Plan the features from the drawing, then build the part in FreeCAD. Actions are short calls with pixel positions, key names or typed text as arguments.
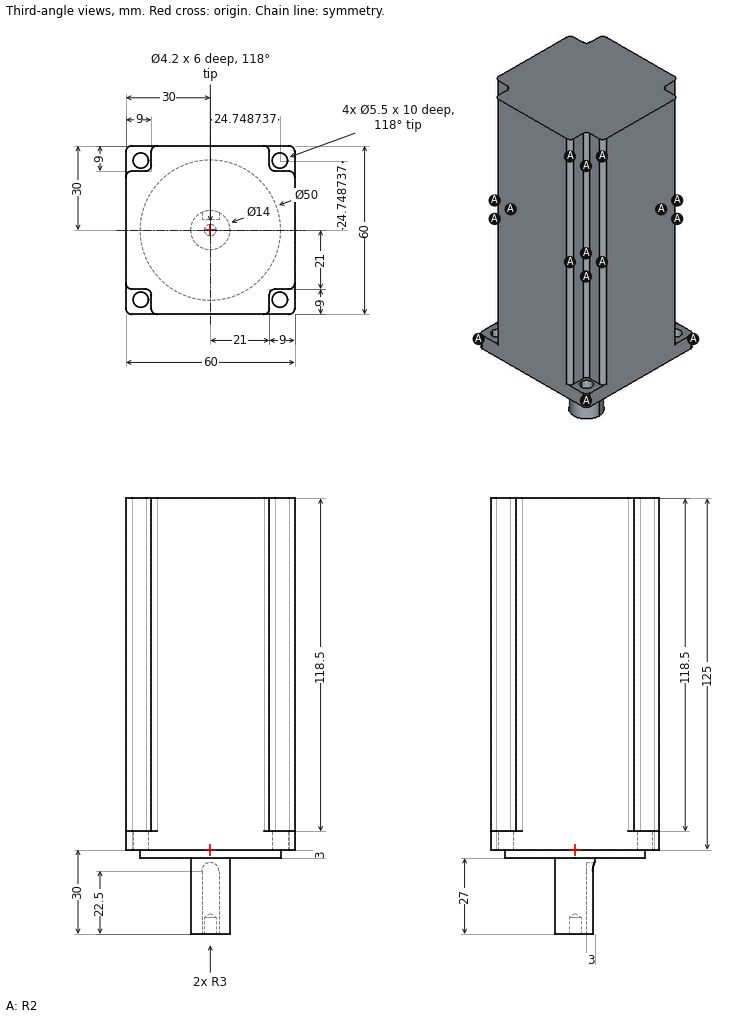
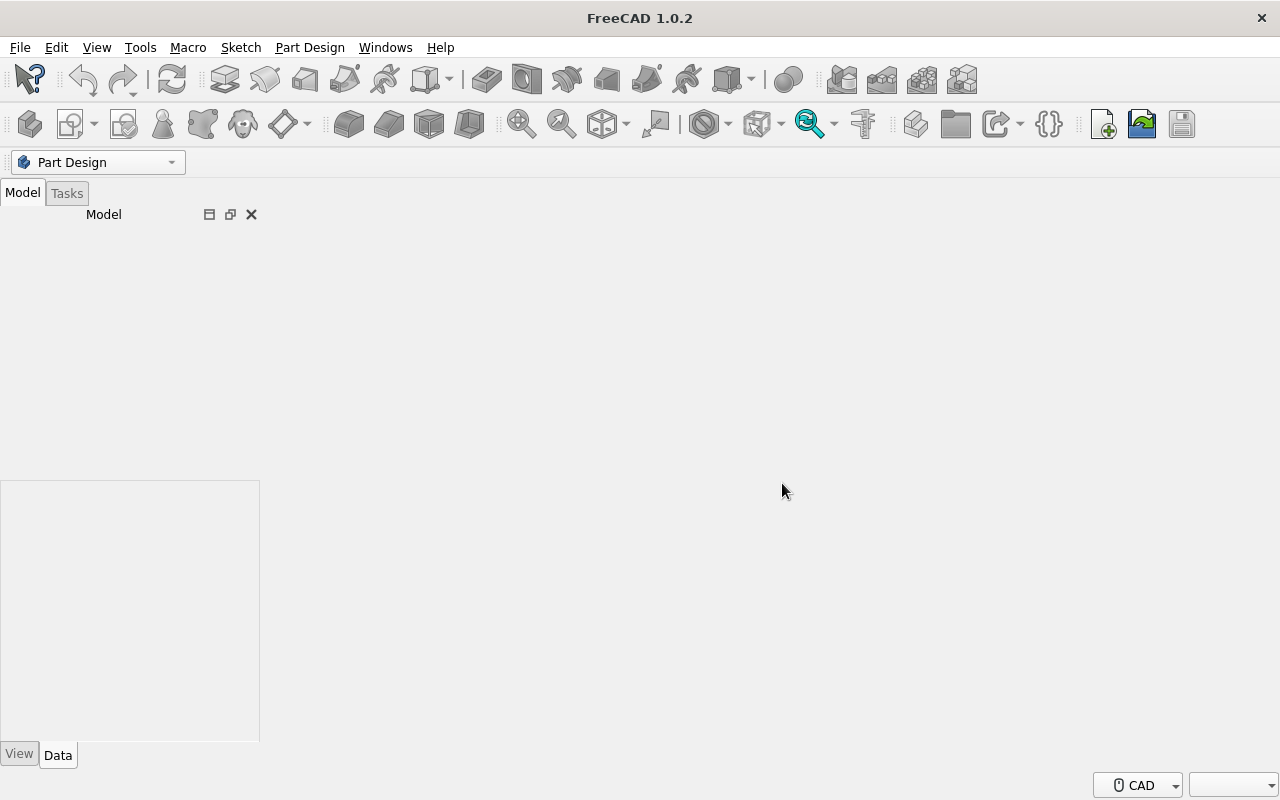
click(1102, 124)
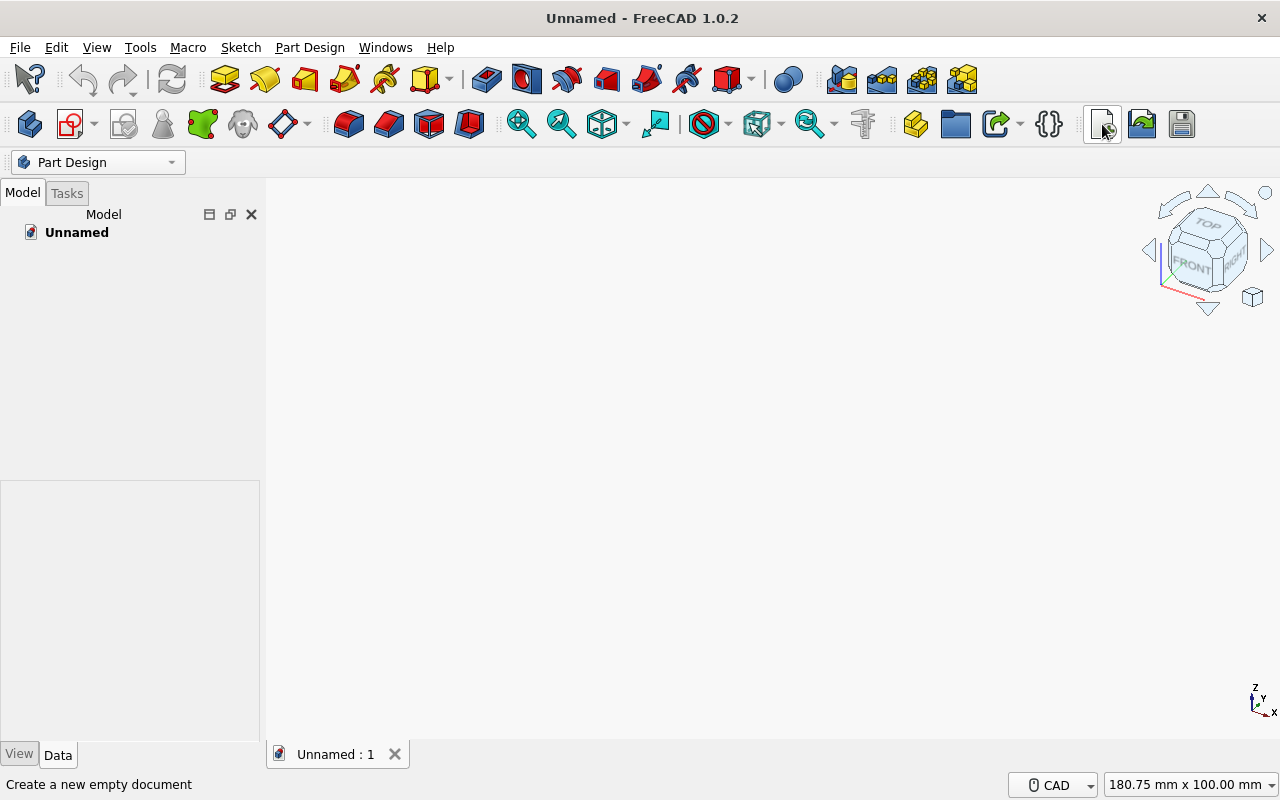
click(70, 124)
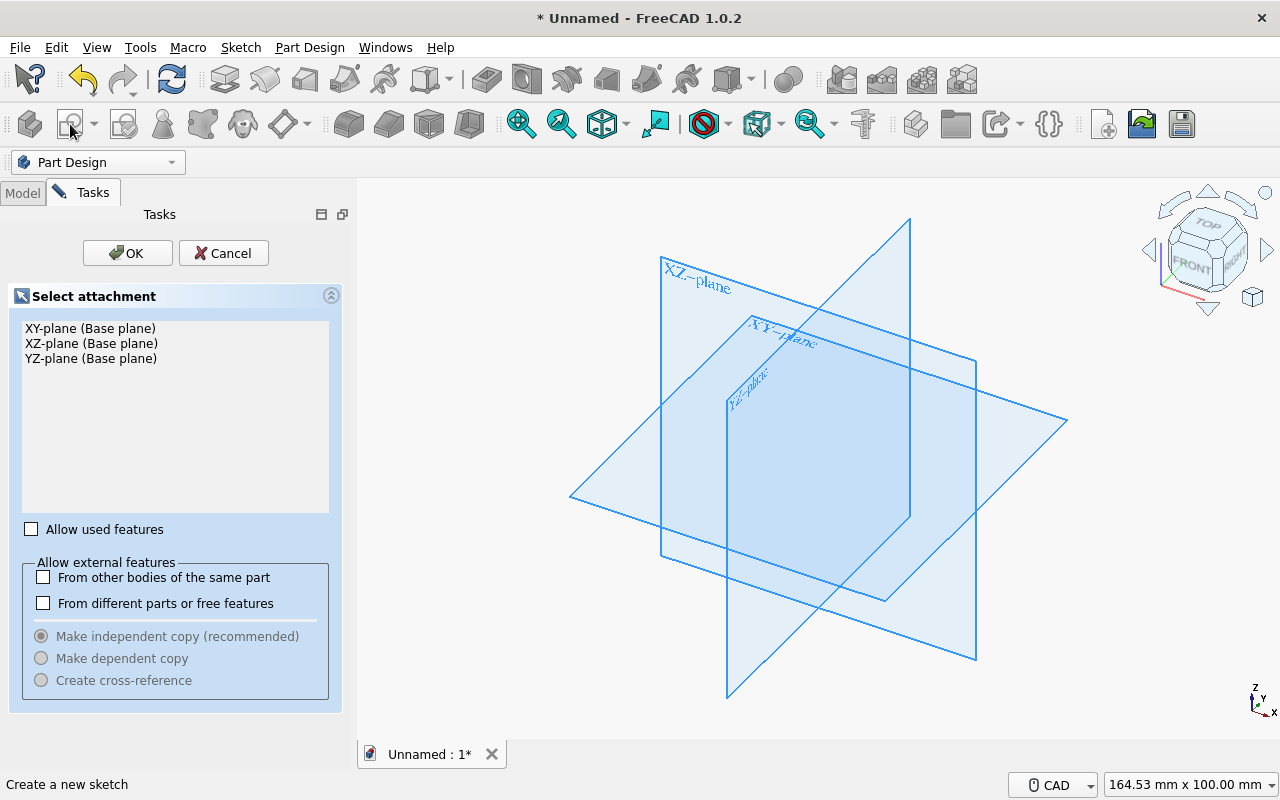
click(82, 328)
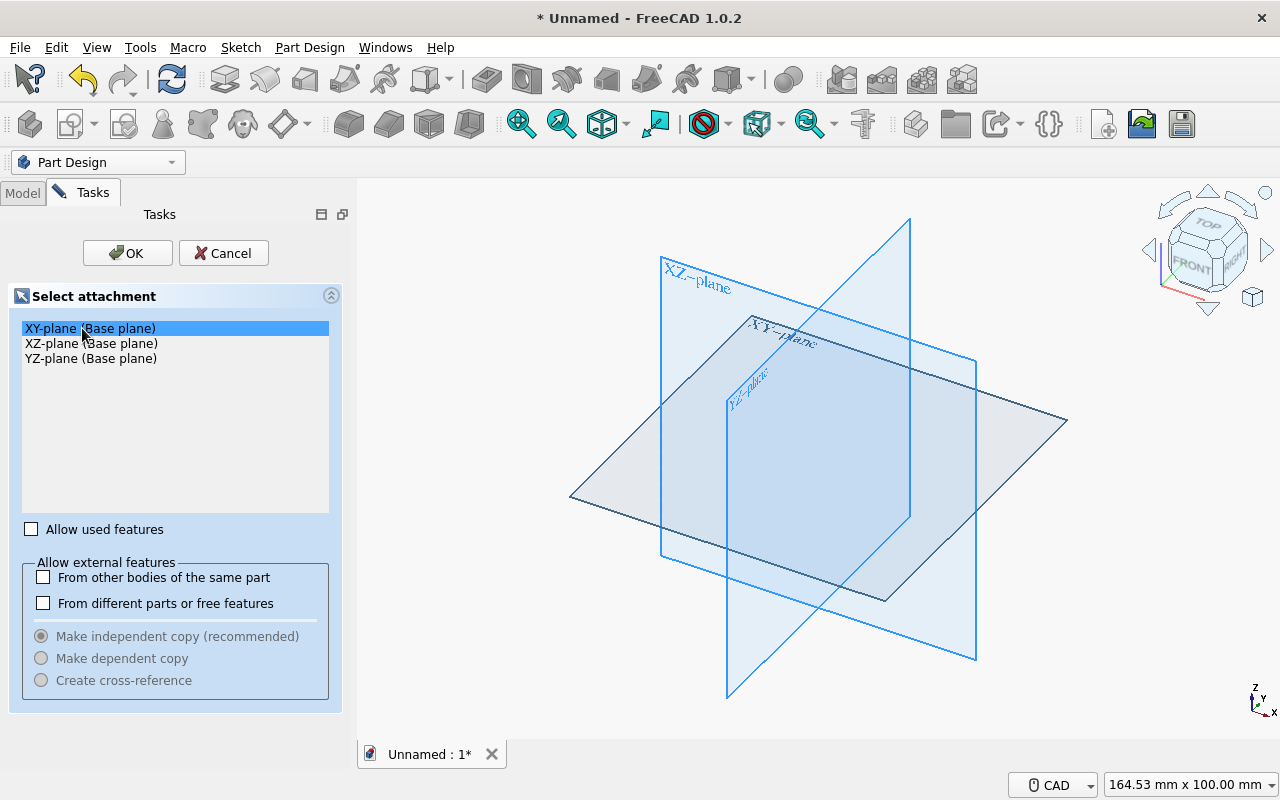
click(128, 253)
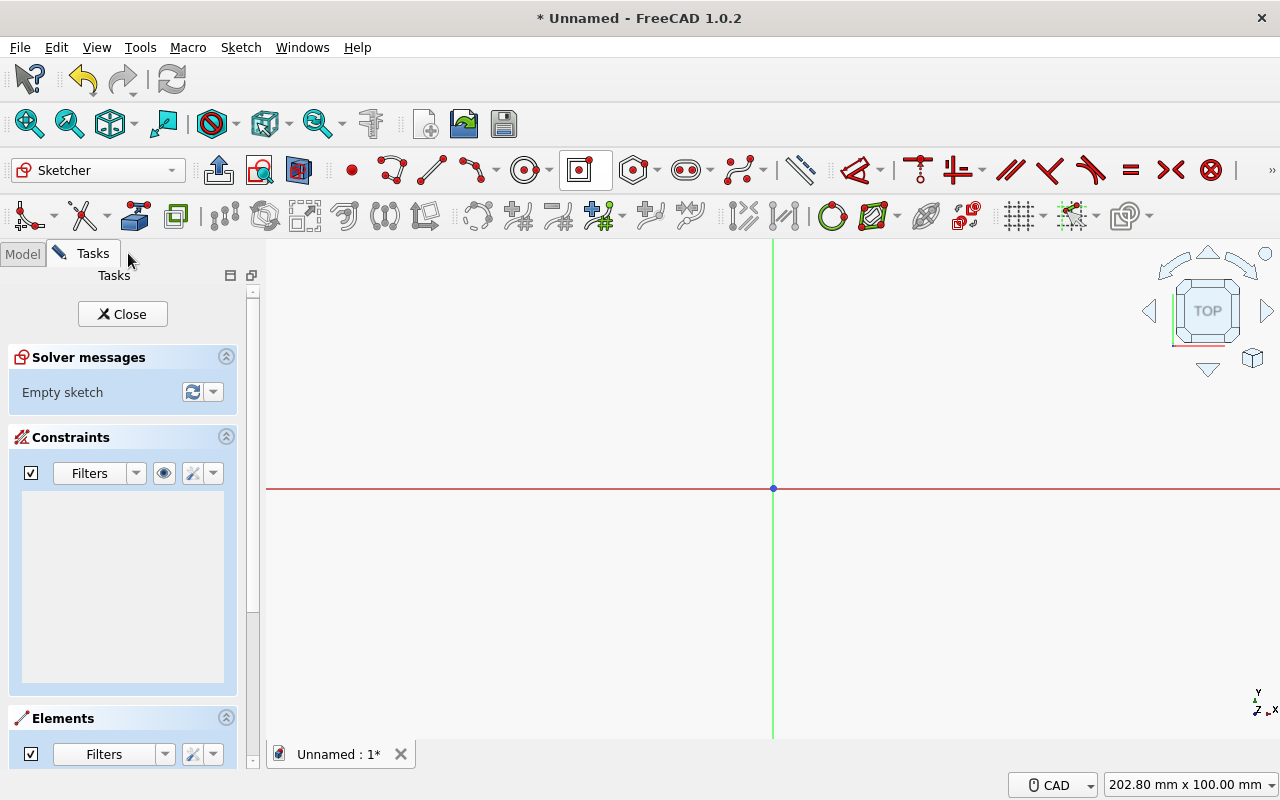
key(g)
key(v)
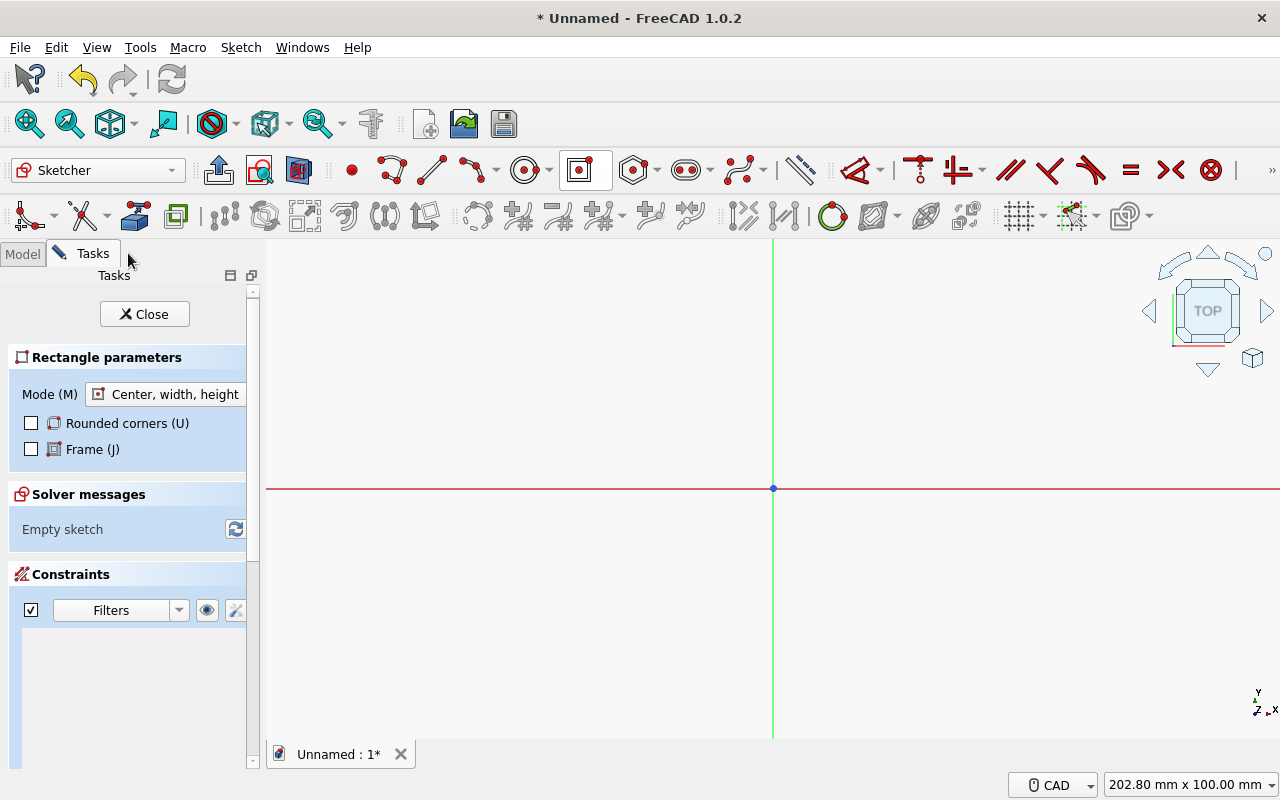
click(773, 489)
move(923, 339)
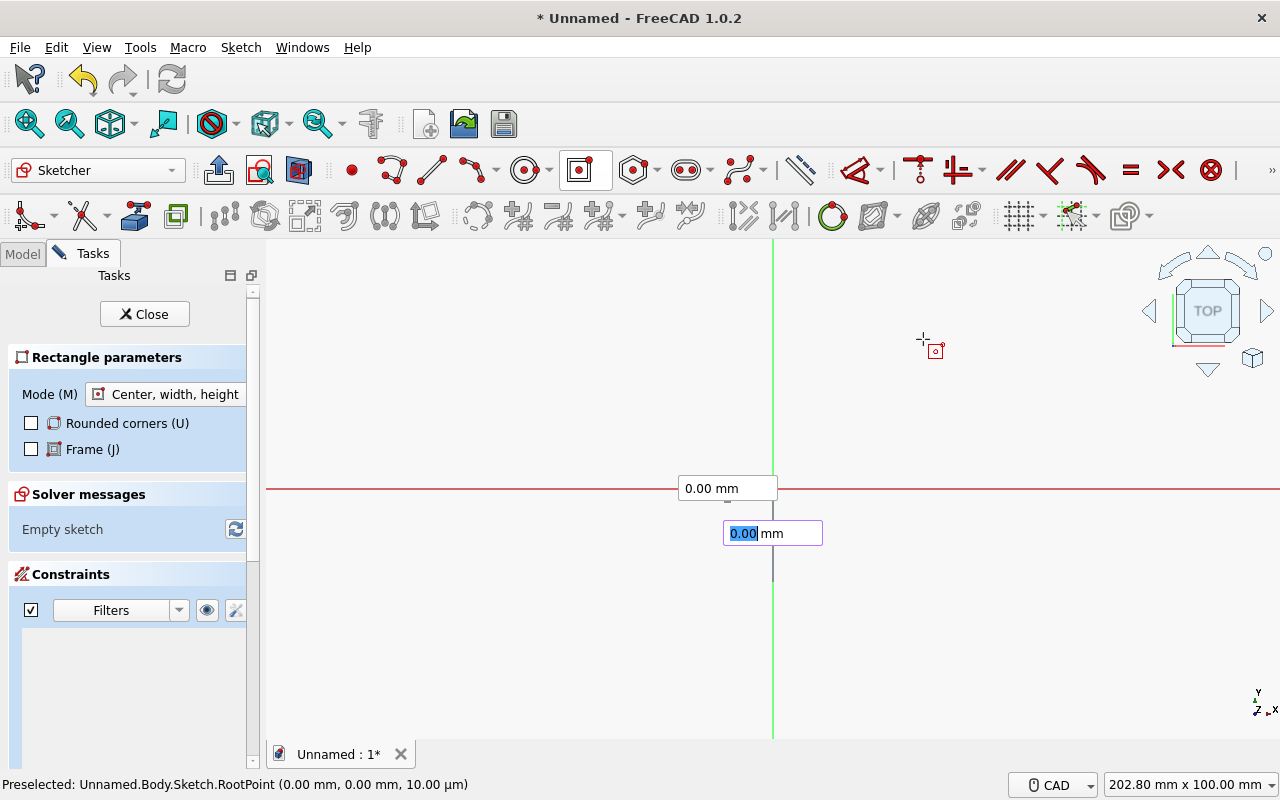
text(60)
key(Tab)
text(60)
key(Return)
key(Escape)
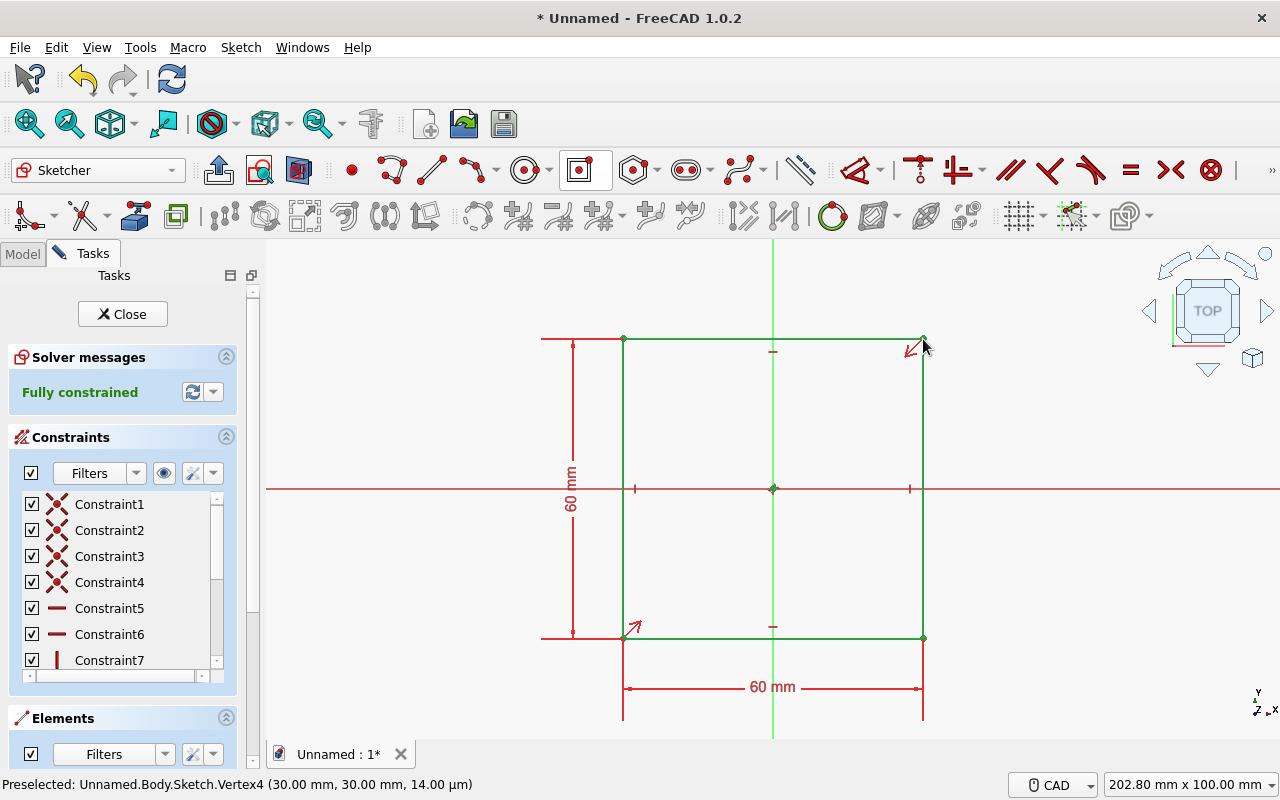
click(123, 314)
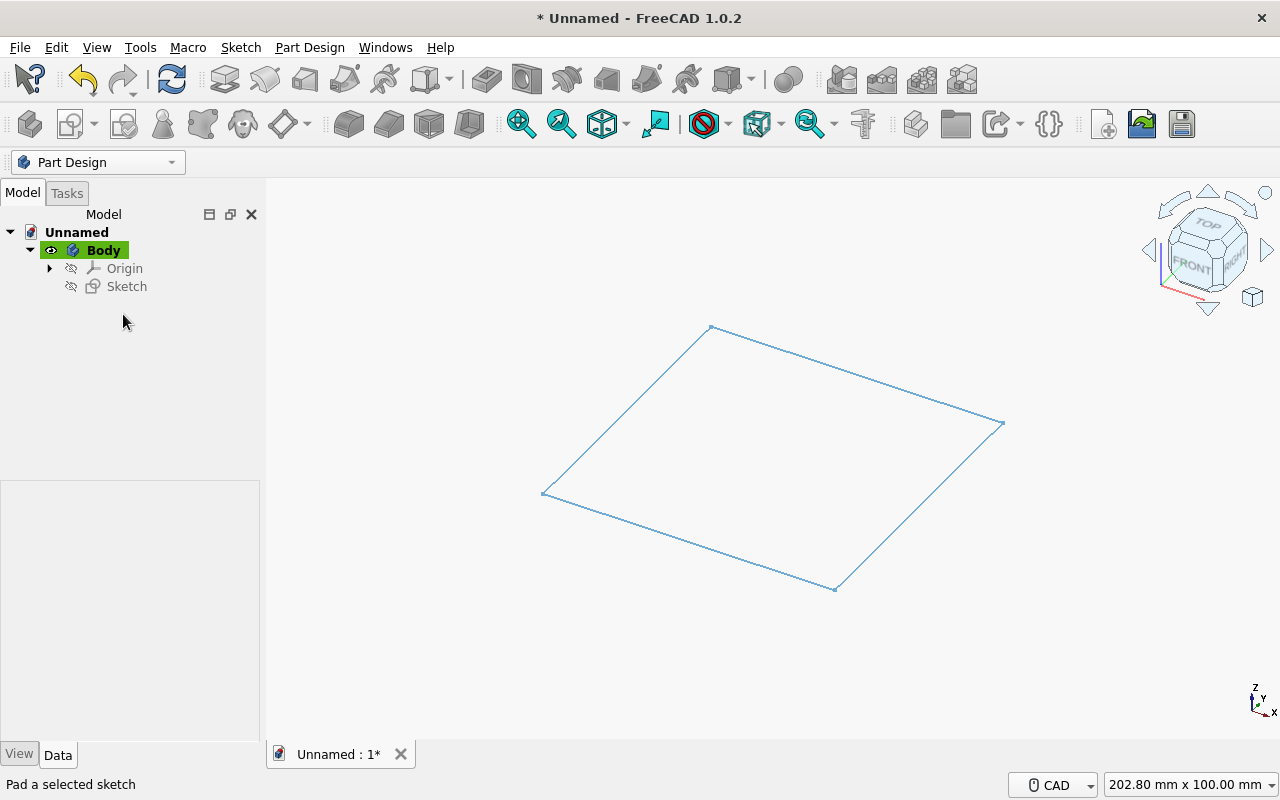
click(226, 80)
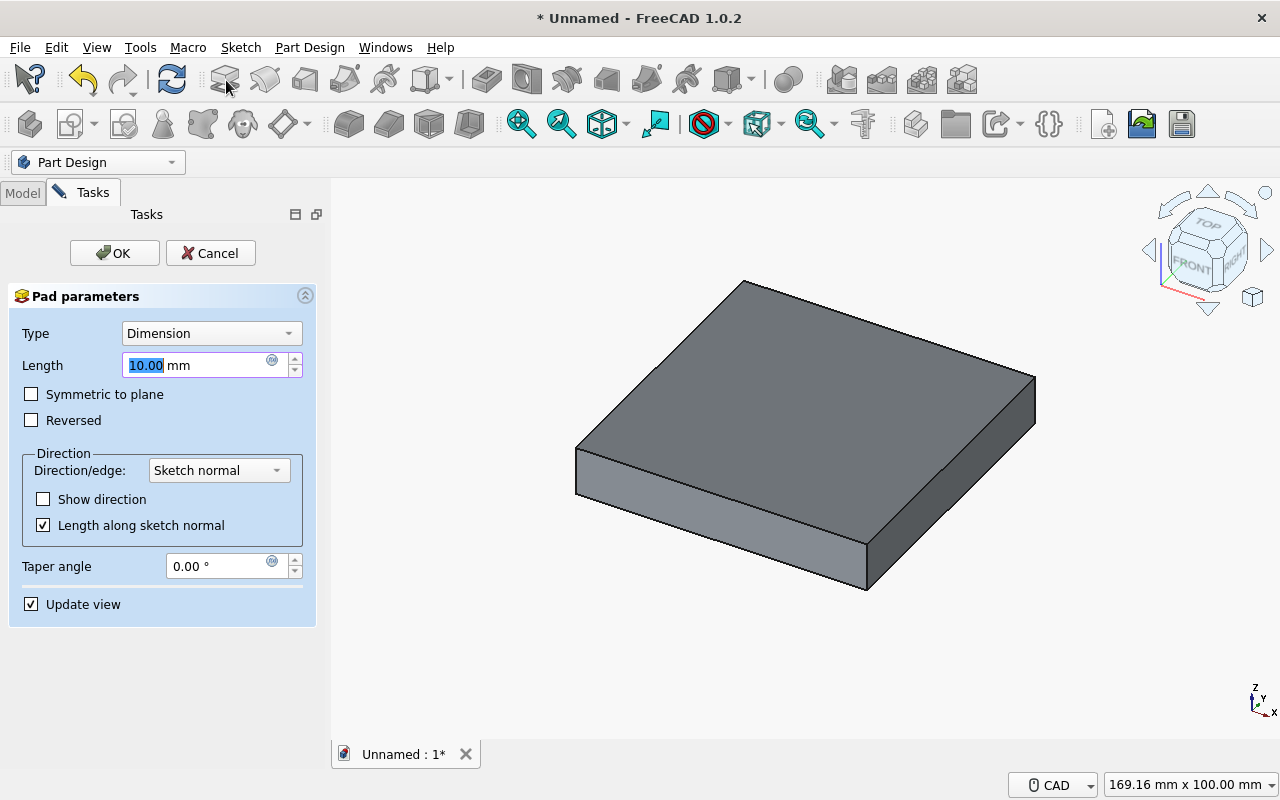
text(125)
key(Tab)